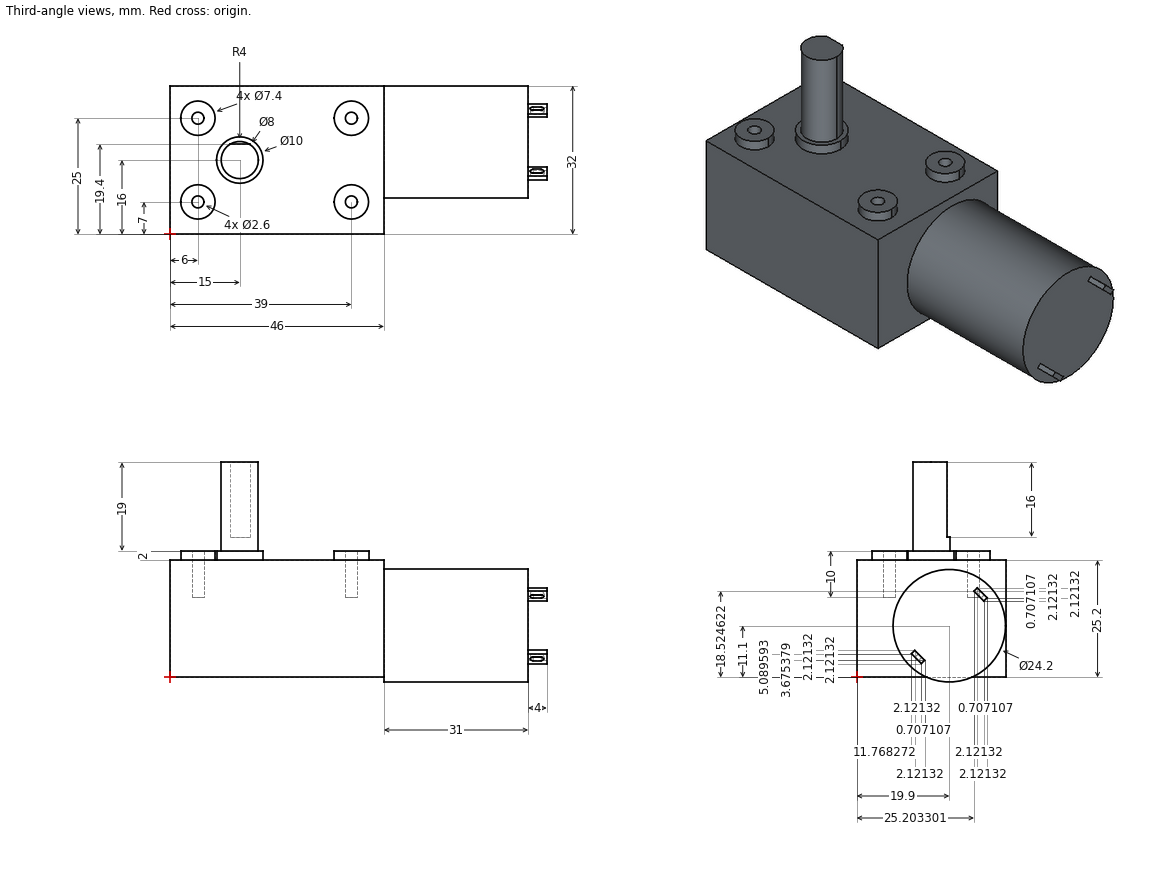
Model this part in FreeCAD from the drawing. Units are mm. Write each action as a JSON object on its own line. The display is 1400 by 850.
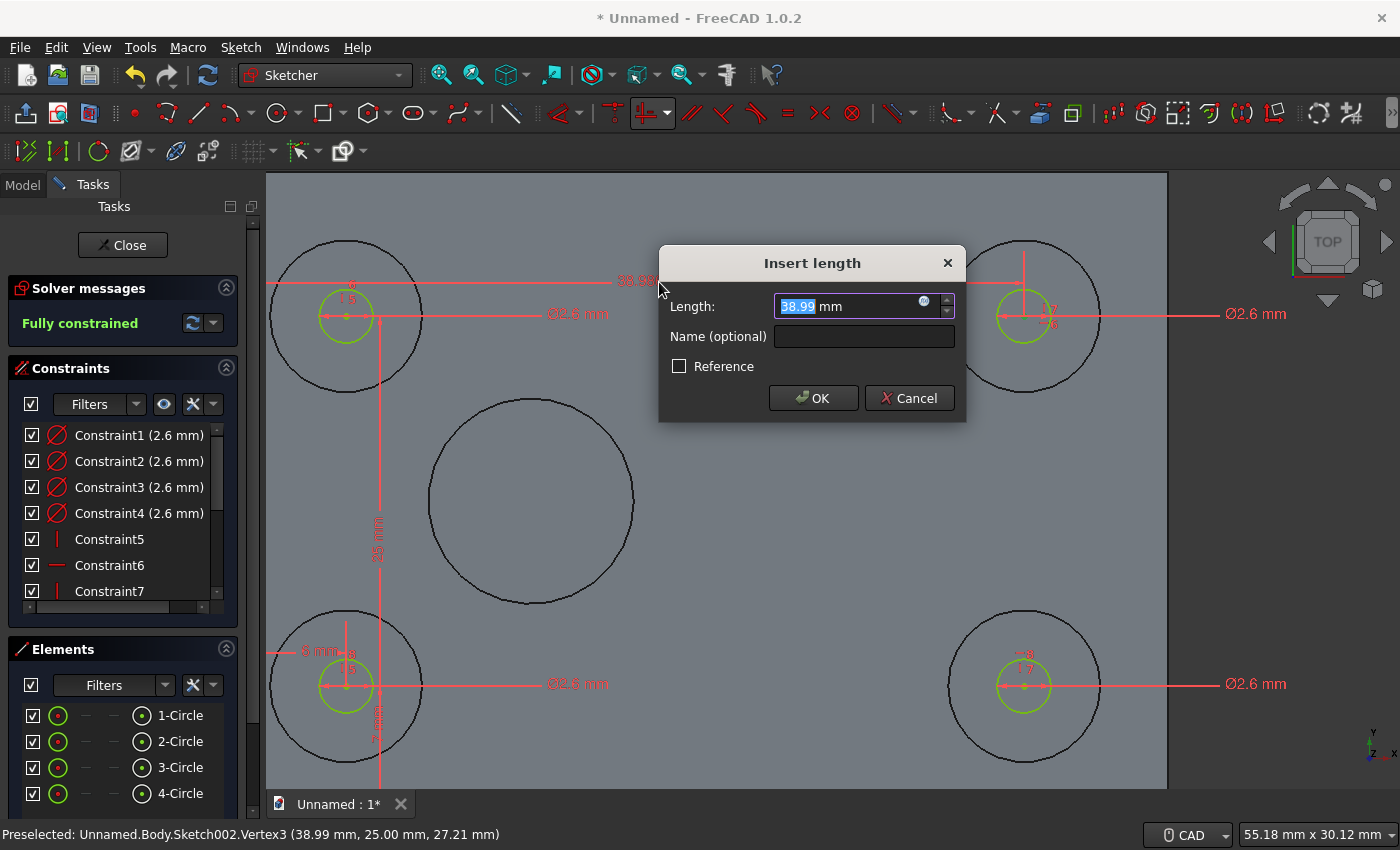
{"action": "type", "text": "39"}
{"action": "key", "text": "Return"}
{"action": "key", "text": "Escape"}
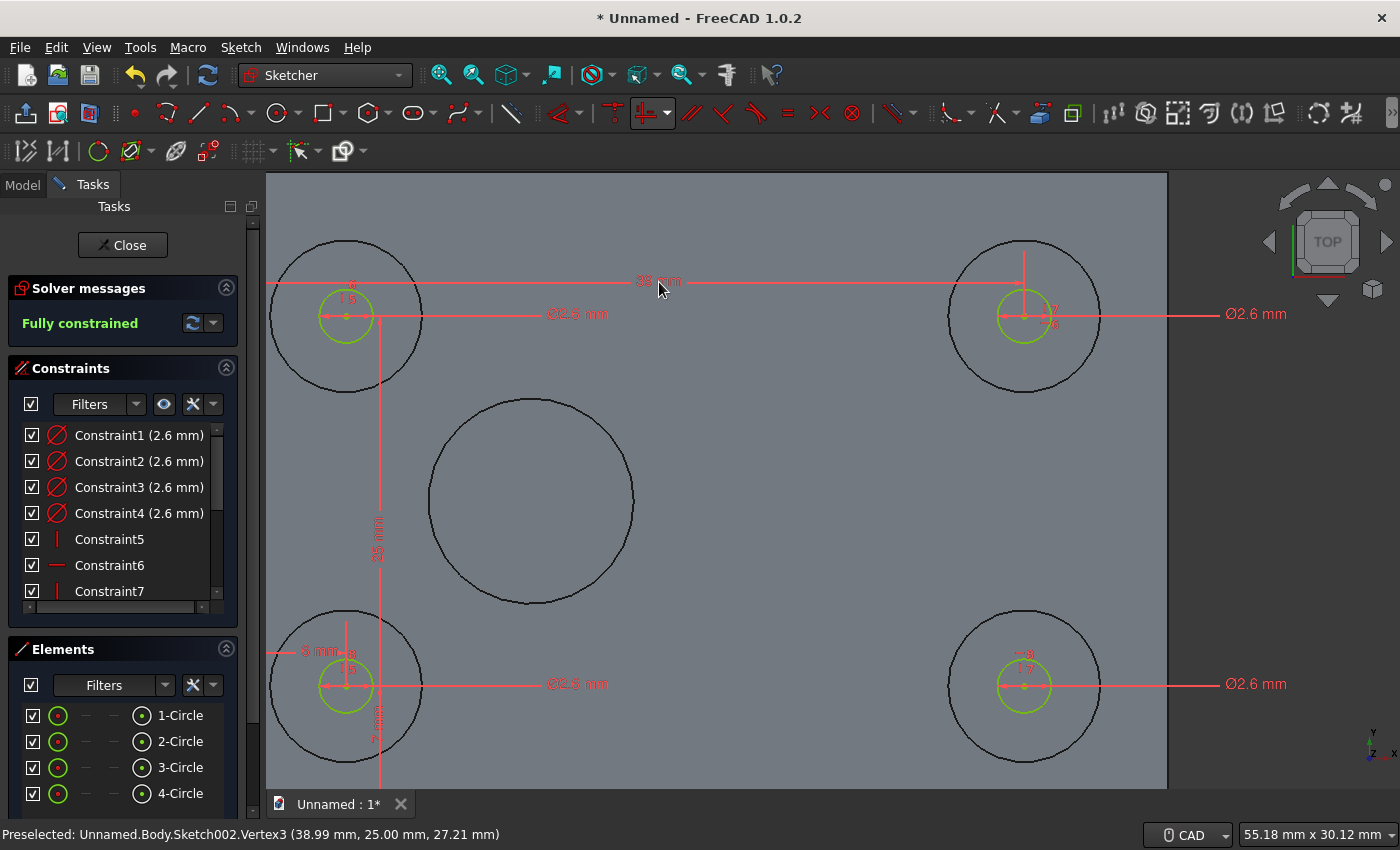
{"action": "left_click", "coordinate": [123, 245]}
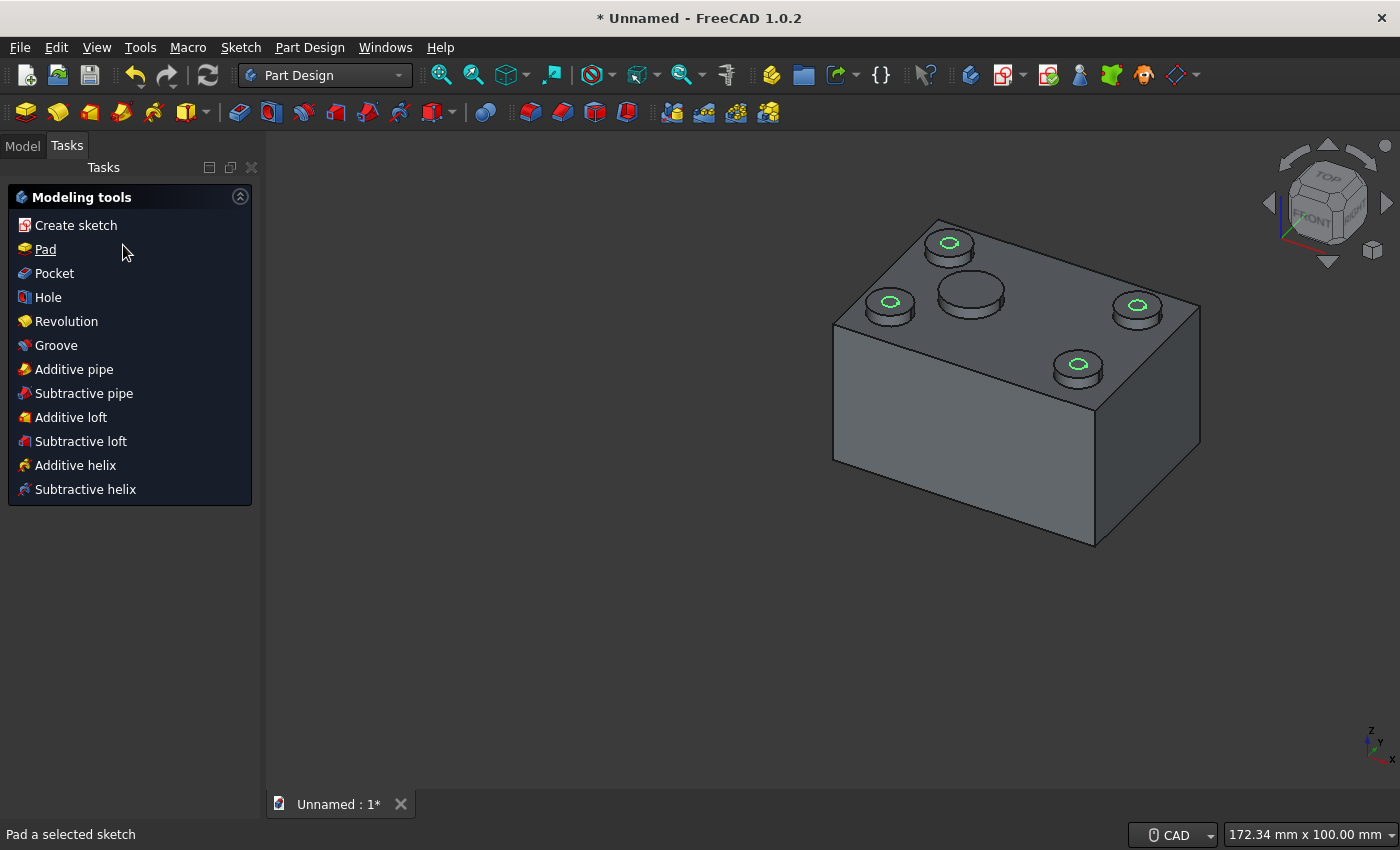
{"action": "left_click", "coordinate": [240, 112]}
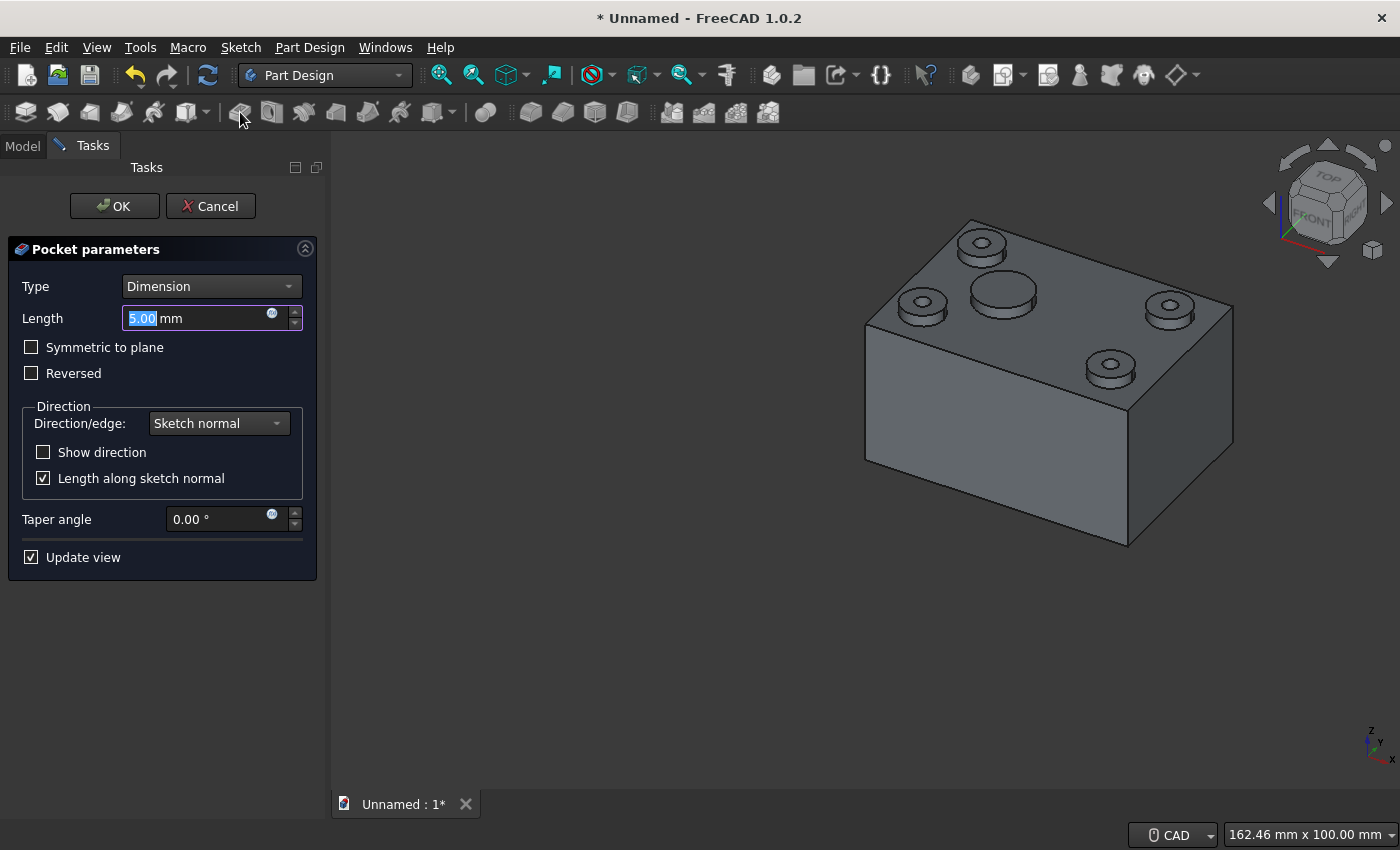
{"action": "type", "text": "10"}
{"action": "key", "text": "Tab"}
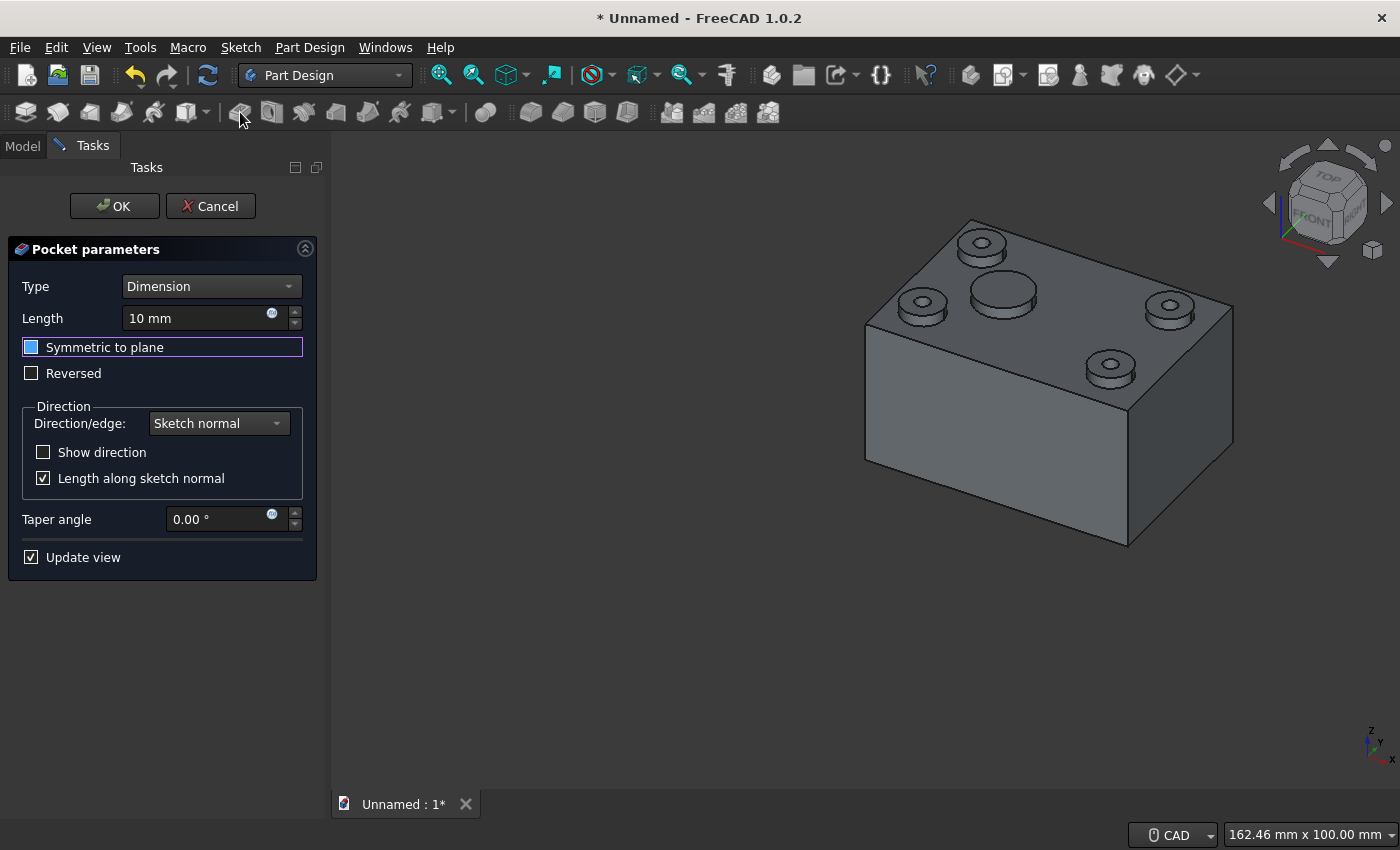
{"action": "left_click", "coordinate": [115, 206]}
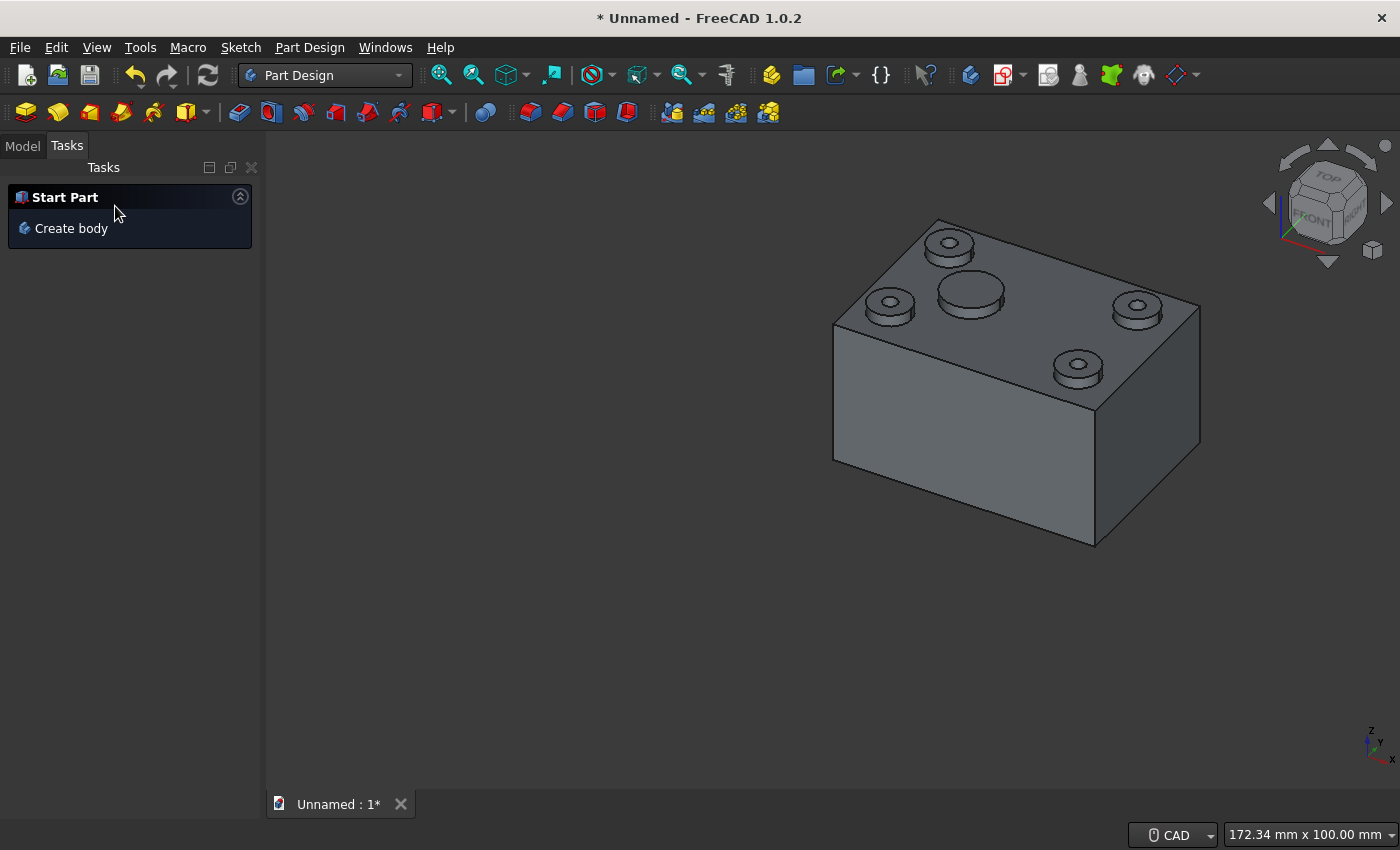
{"action": "left_click", "coordinate": [971, 288]}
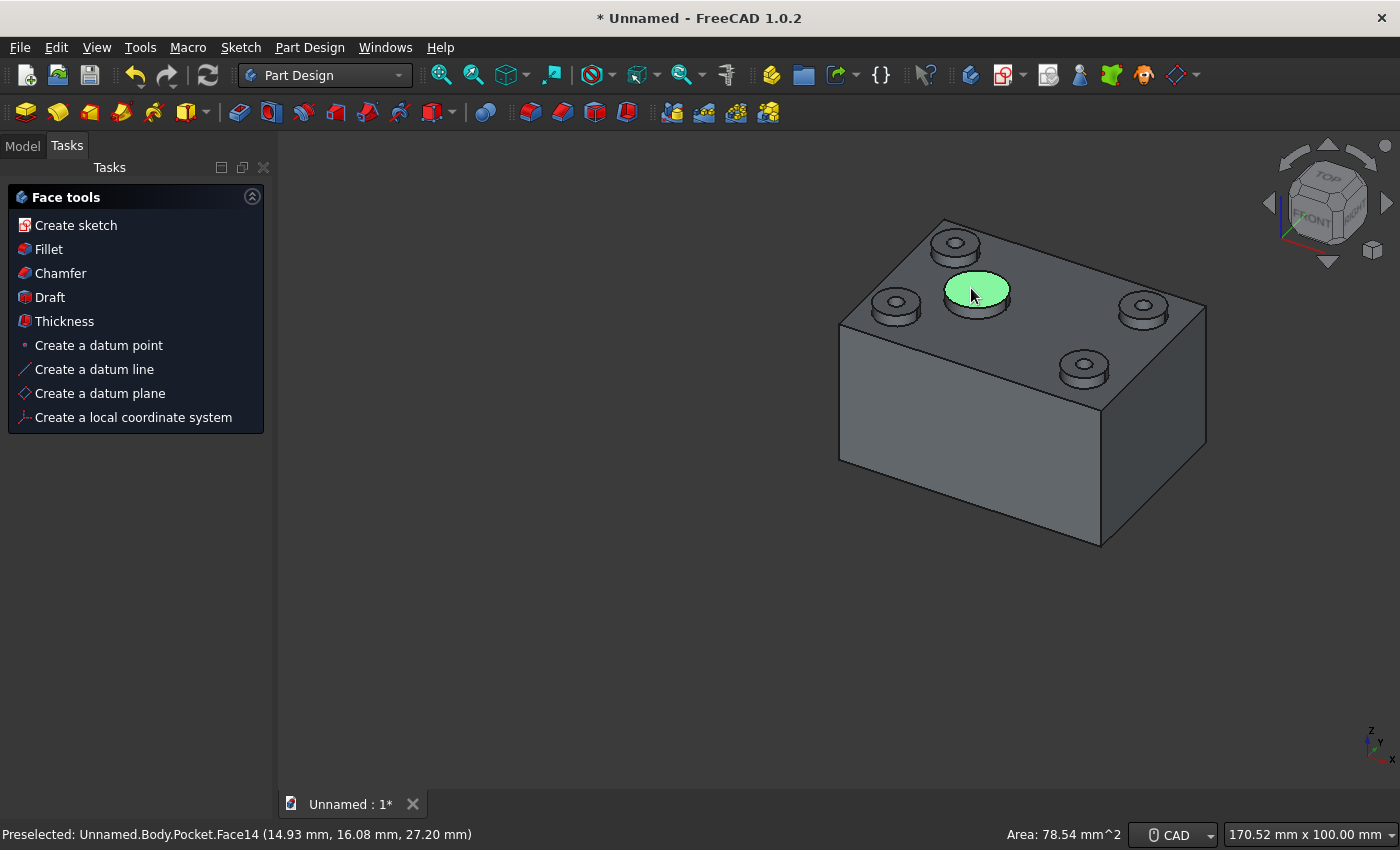
{"action": "left_click", "coordinate": [1004, 76]}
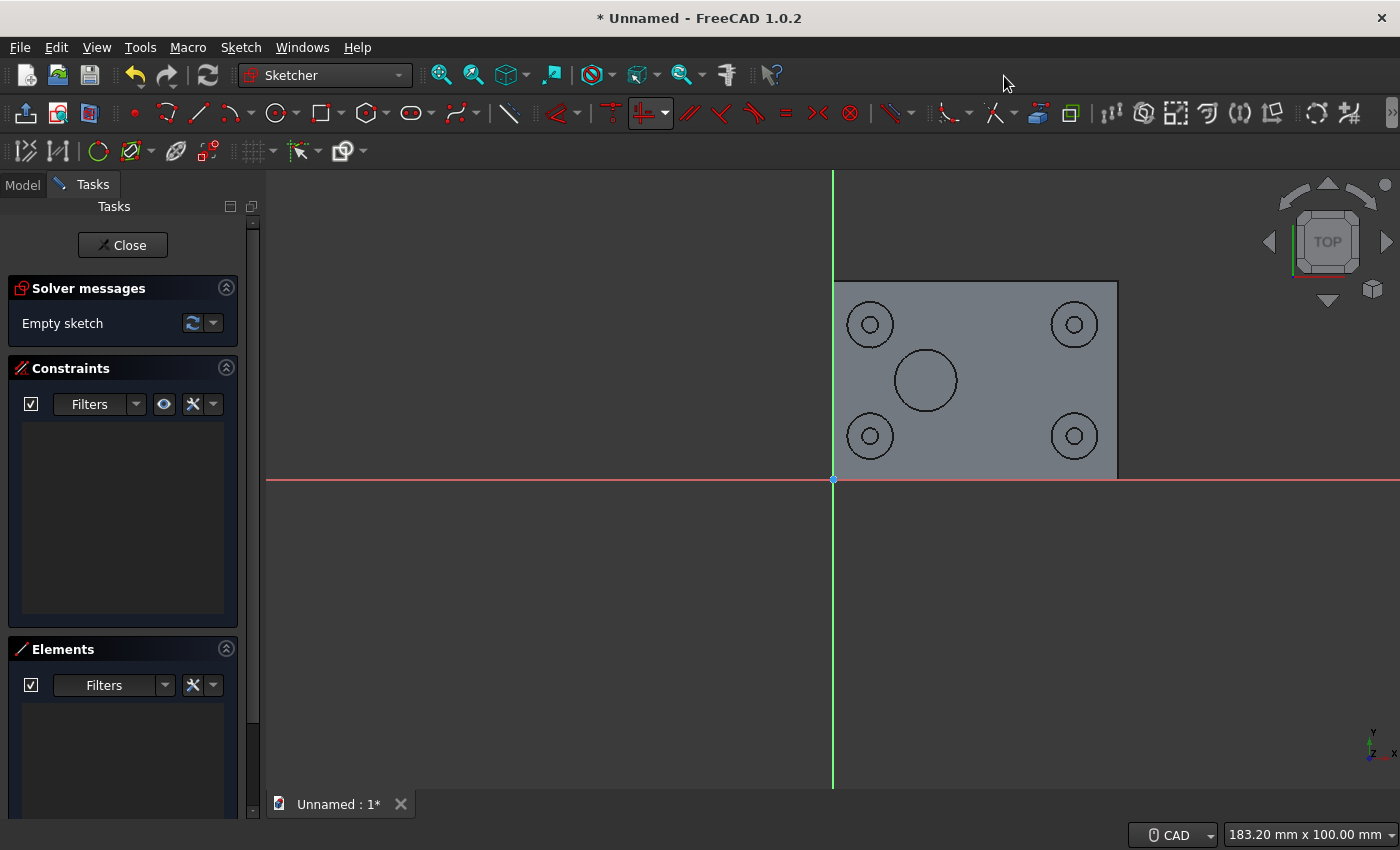
{"action": "scroll", "coordinate": [951, 365], "scroll_direction": "up", "scroll_amount": 10}